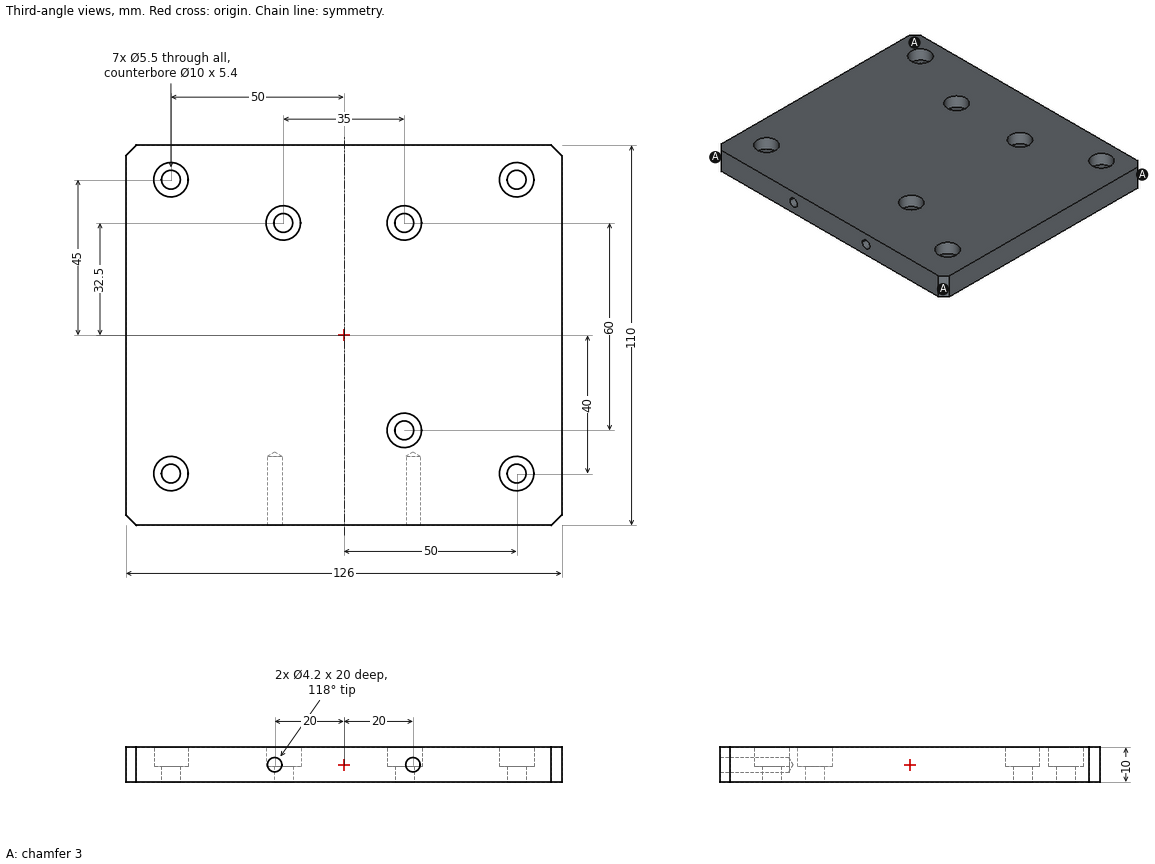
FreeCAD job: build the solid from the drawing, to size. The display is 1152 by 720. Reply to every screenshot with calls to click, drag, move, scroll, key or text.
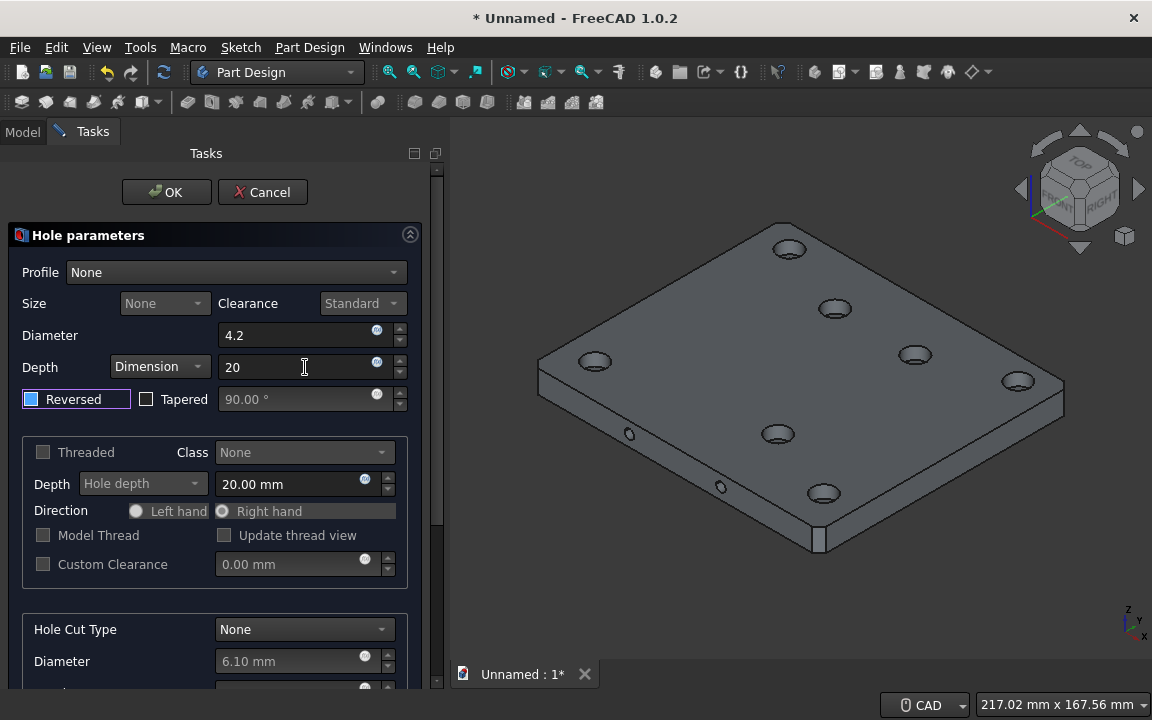
click(167, 192)